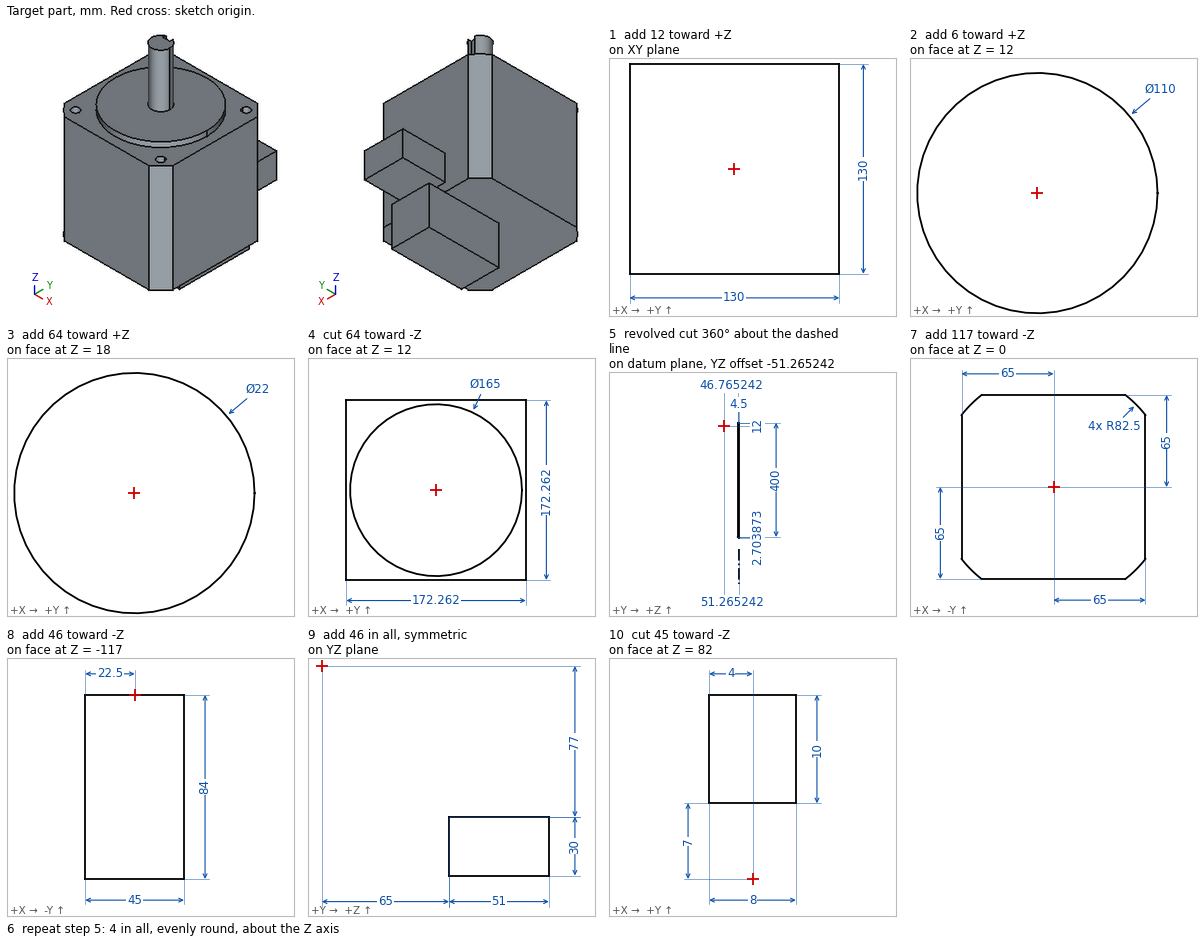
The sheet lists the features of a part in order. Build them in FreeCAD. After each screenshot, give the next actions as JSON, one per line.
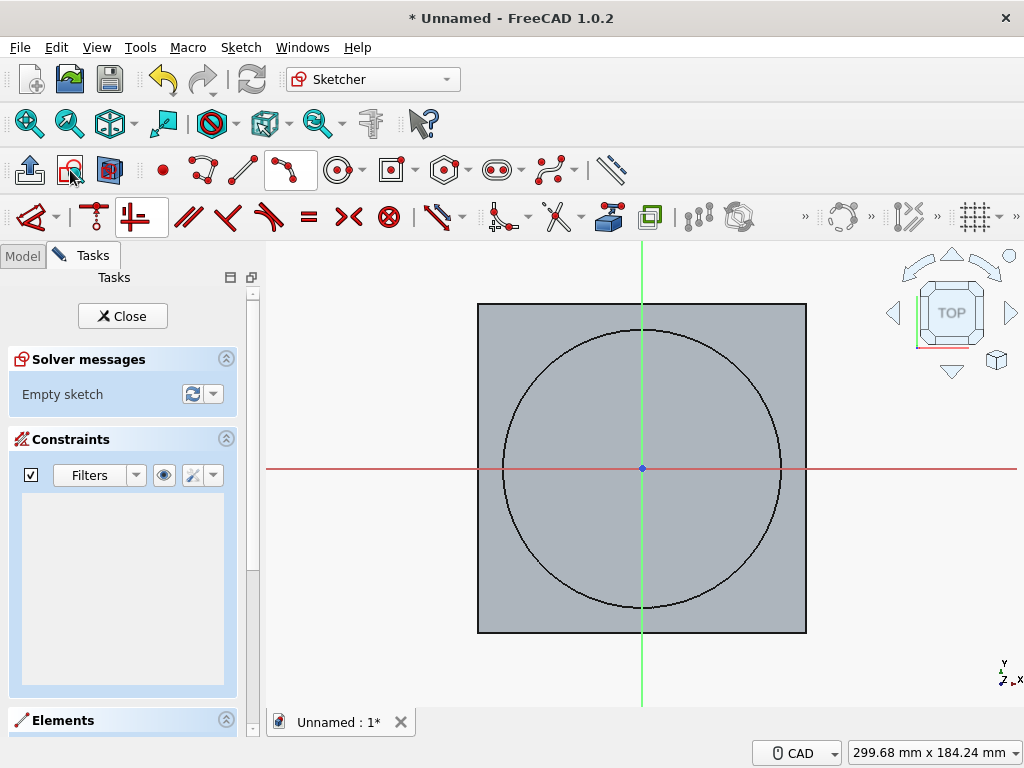
{"action": "scroll", "coordinate": [659, 468], "scroll_direction": "up", "scroll_amount": 8}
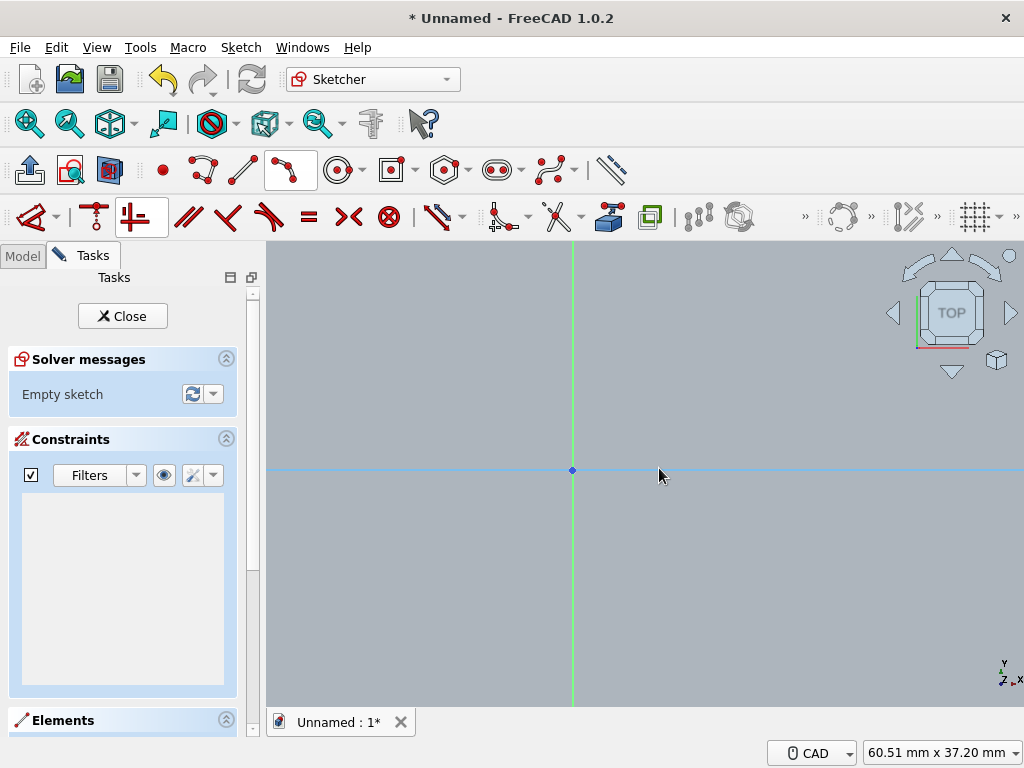
{"action": "left_click", "coordinate": [338, 170]}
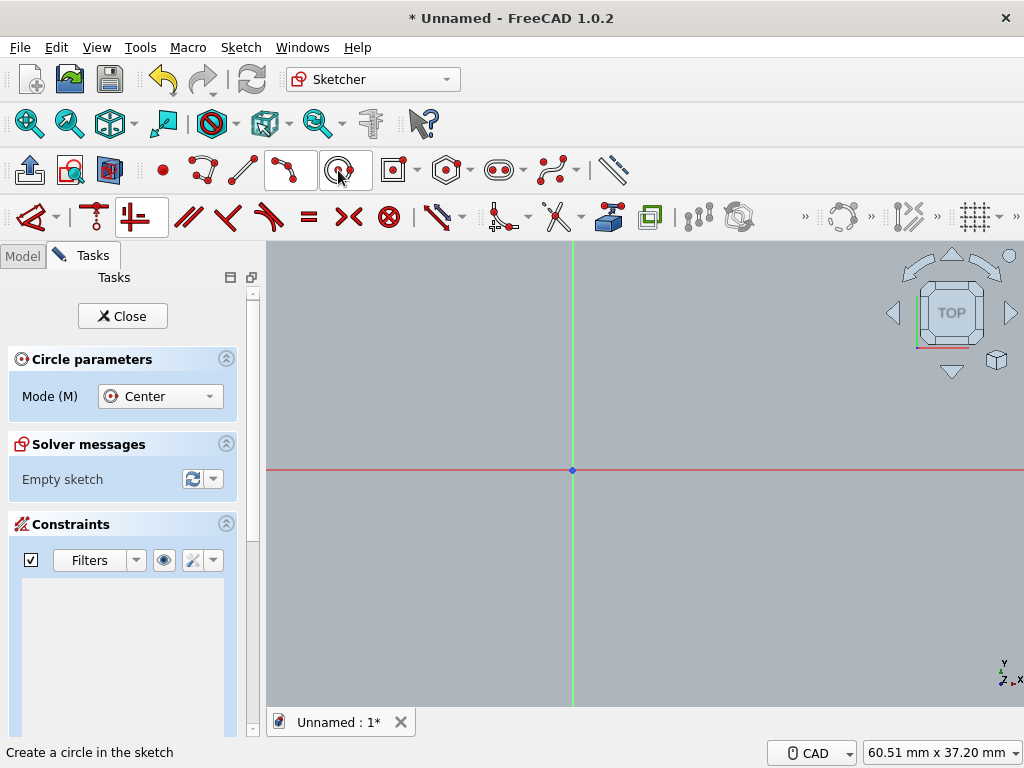
{"action": "left_click", "coordinate": [573, 470]}
{"action": "mouse_move", "coordinate": [670, 373]}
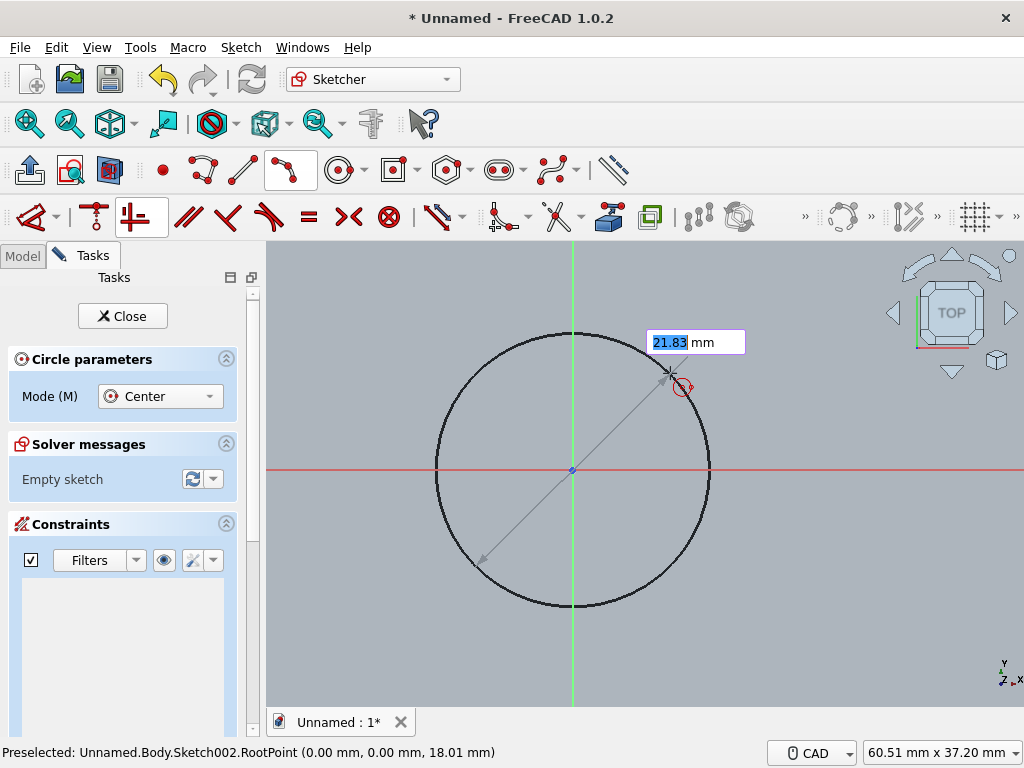
{"action": "type", "text": "22"}
{"action": "key", "text": "Return"}
{"action": "key", "text": "Escape"}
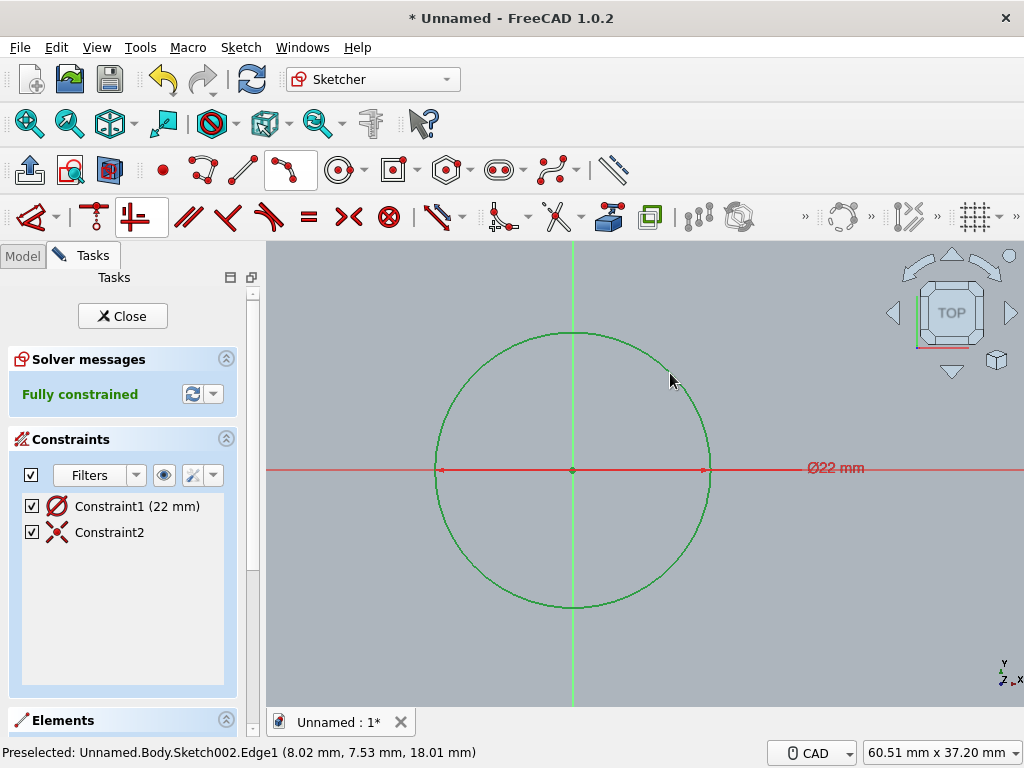
{"action": "left_click", "coordinate": [123, 316]}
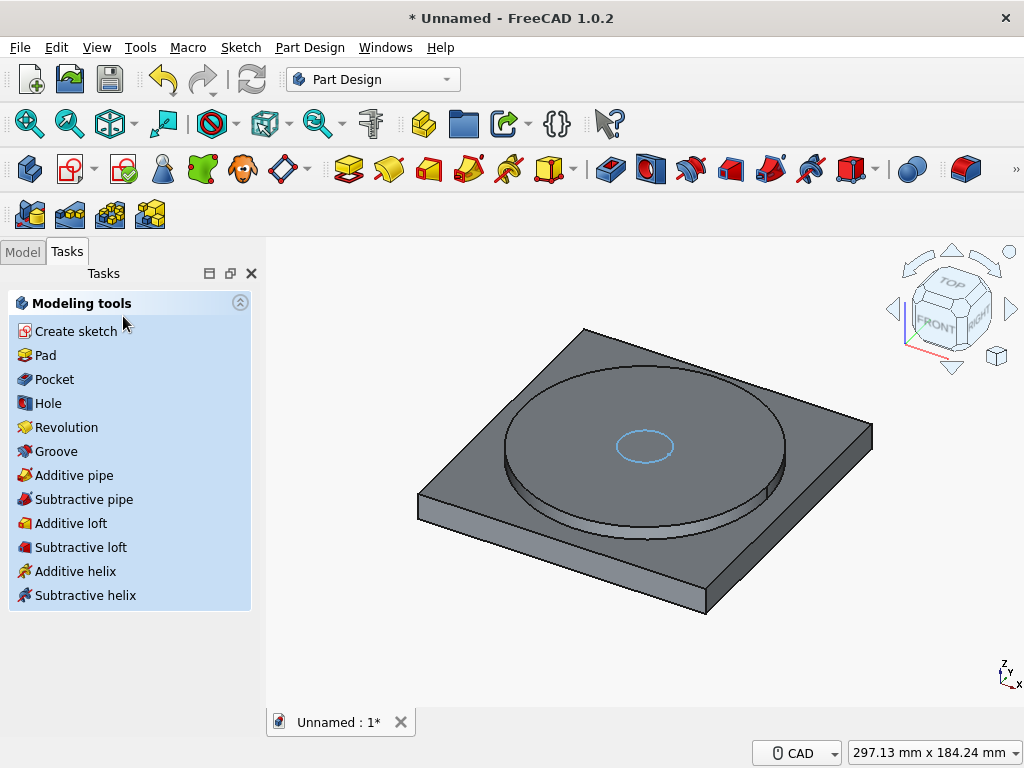
{"action": "left_click", "coordinate": [350, 170]}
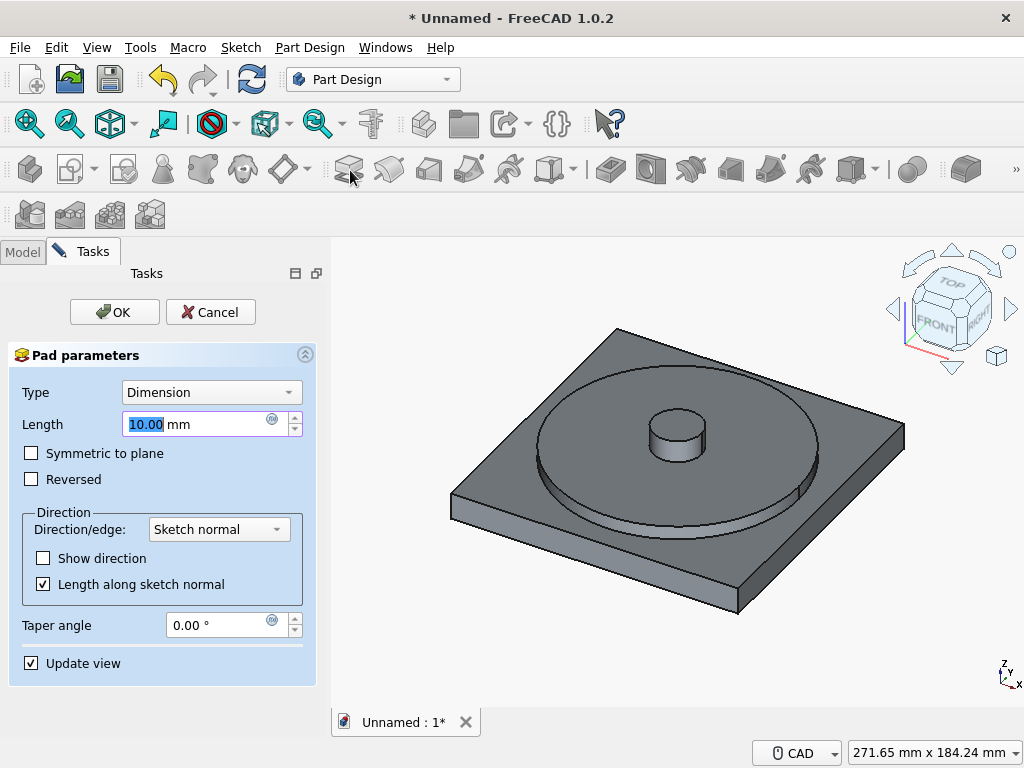
{"action": "type", "text": "64"}
{"action": "key", "text": "Tab"}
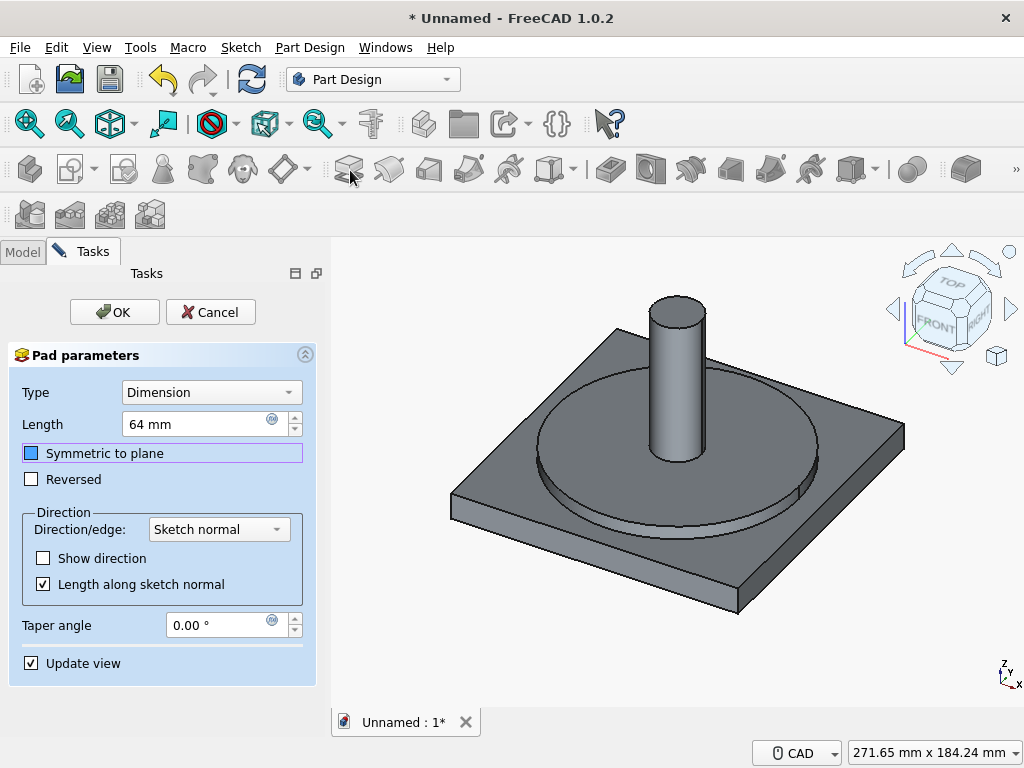
{"action": "left_click", "coordinate": [115, 312]}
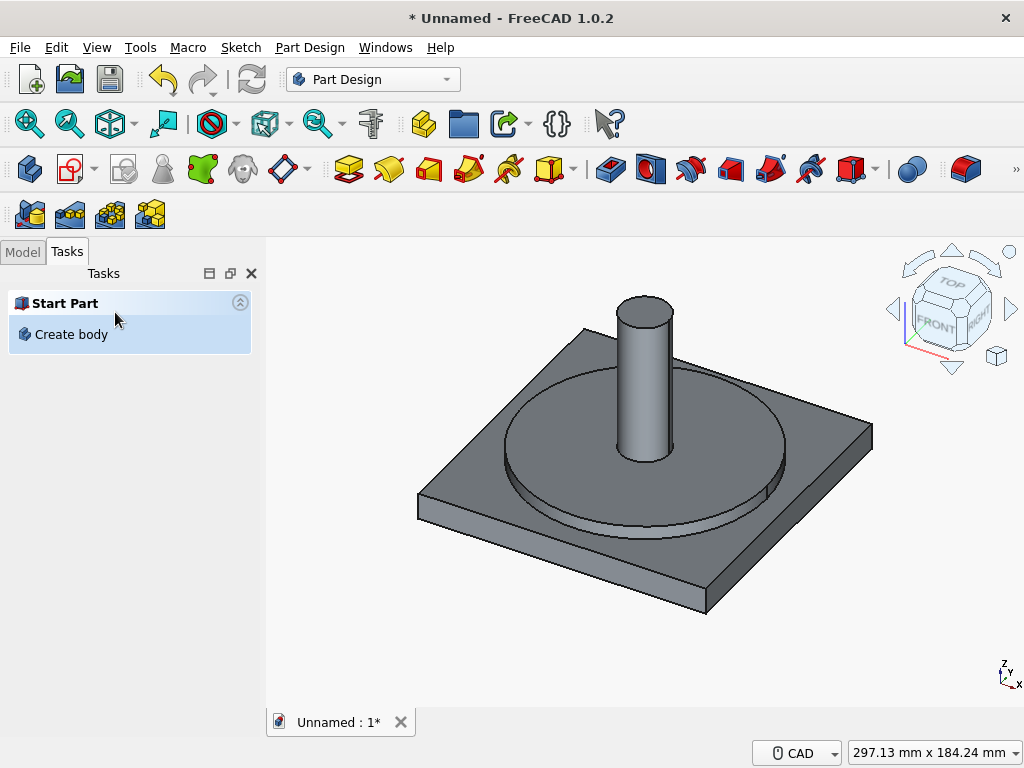
{"action": "left_click", "coordinate": [30, 124]}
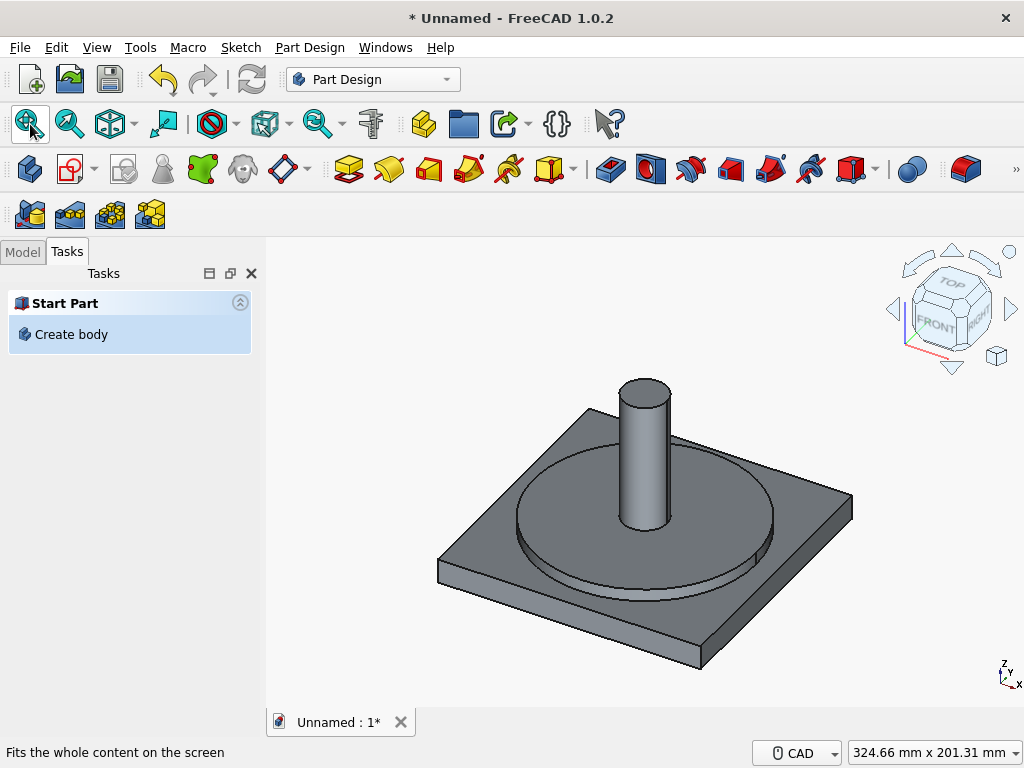
{"action": "left_click", "coordinate": [823, 499]}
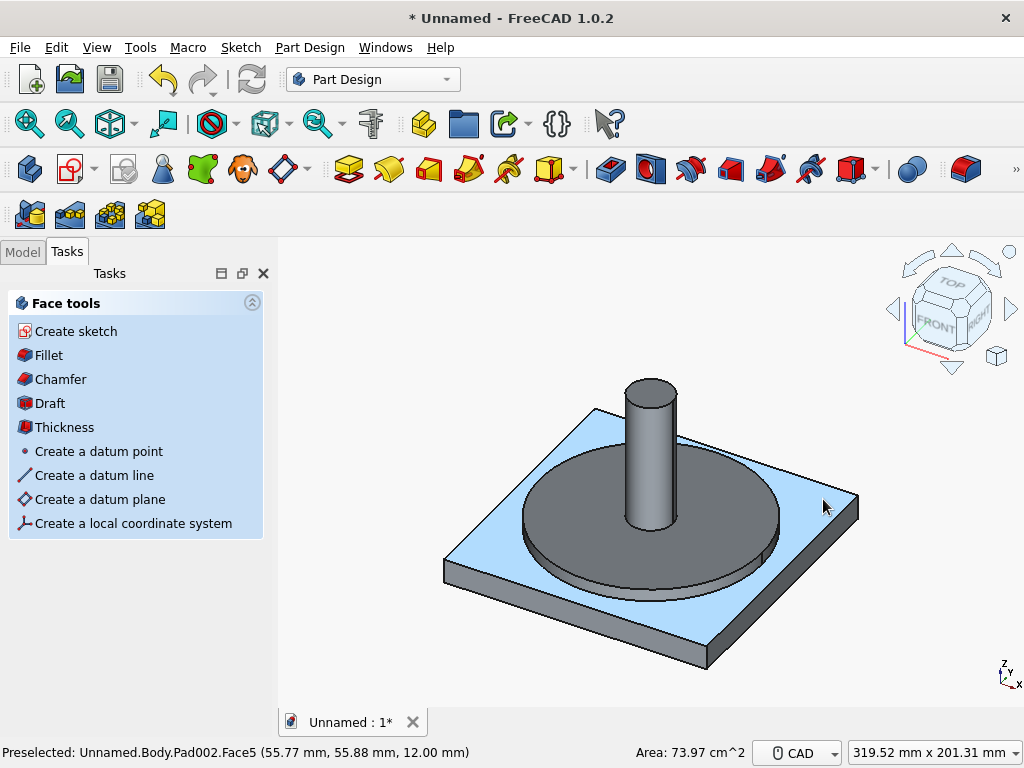
{"action": "left_click", "coordinate": [70, 170]}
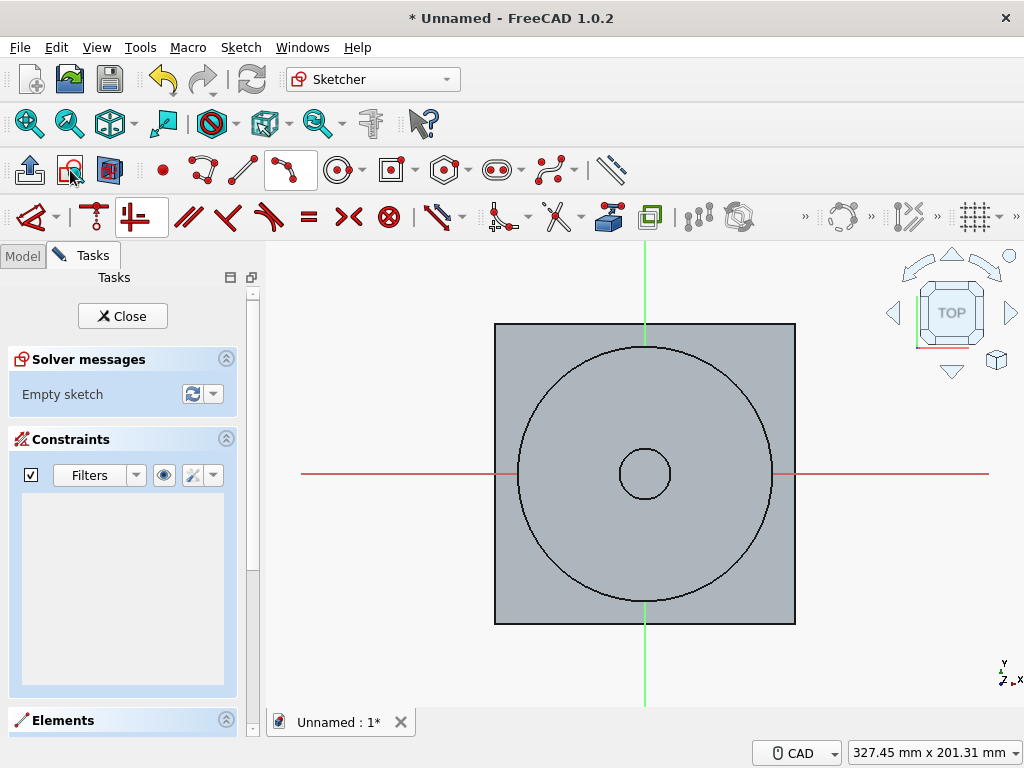
{"action": "scroll", "coordinate": [437, 474], "scroll_direction": "down", "scroll_amount": 2}